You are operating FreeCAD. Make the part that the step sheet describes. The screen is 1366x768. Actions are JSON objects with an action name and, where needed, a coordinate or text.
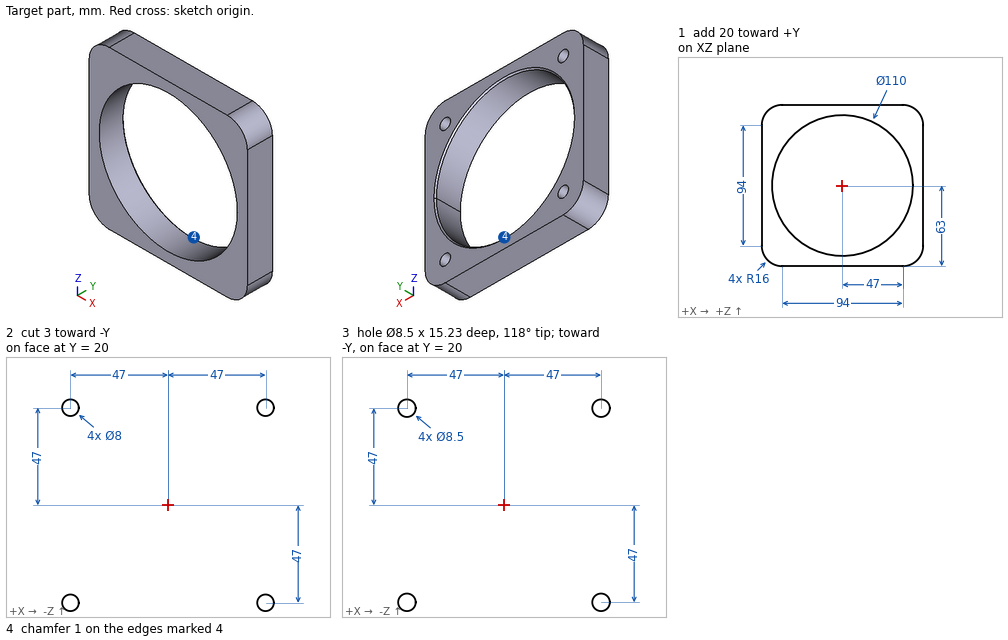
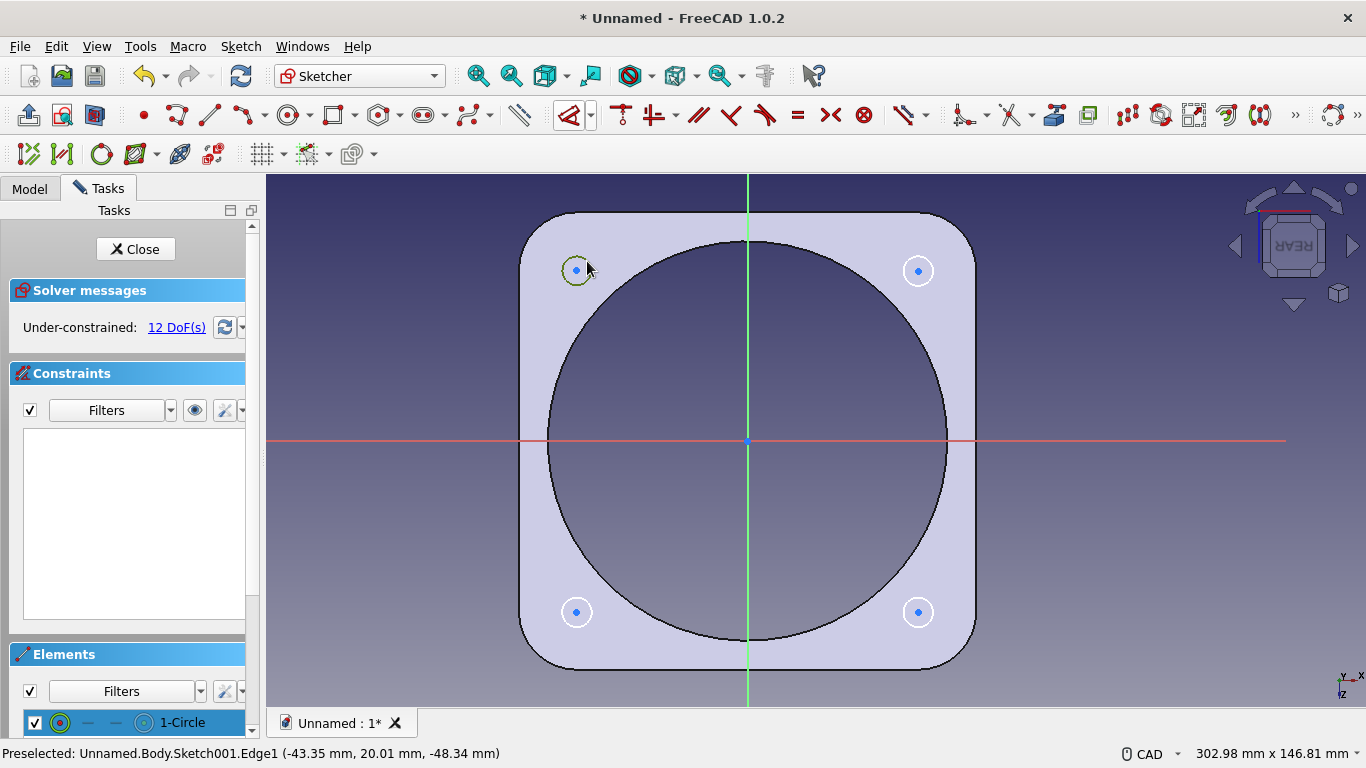
{"action": "left_click", "coordinate": [929, 261]}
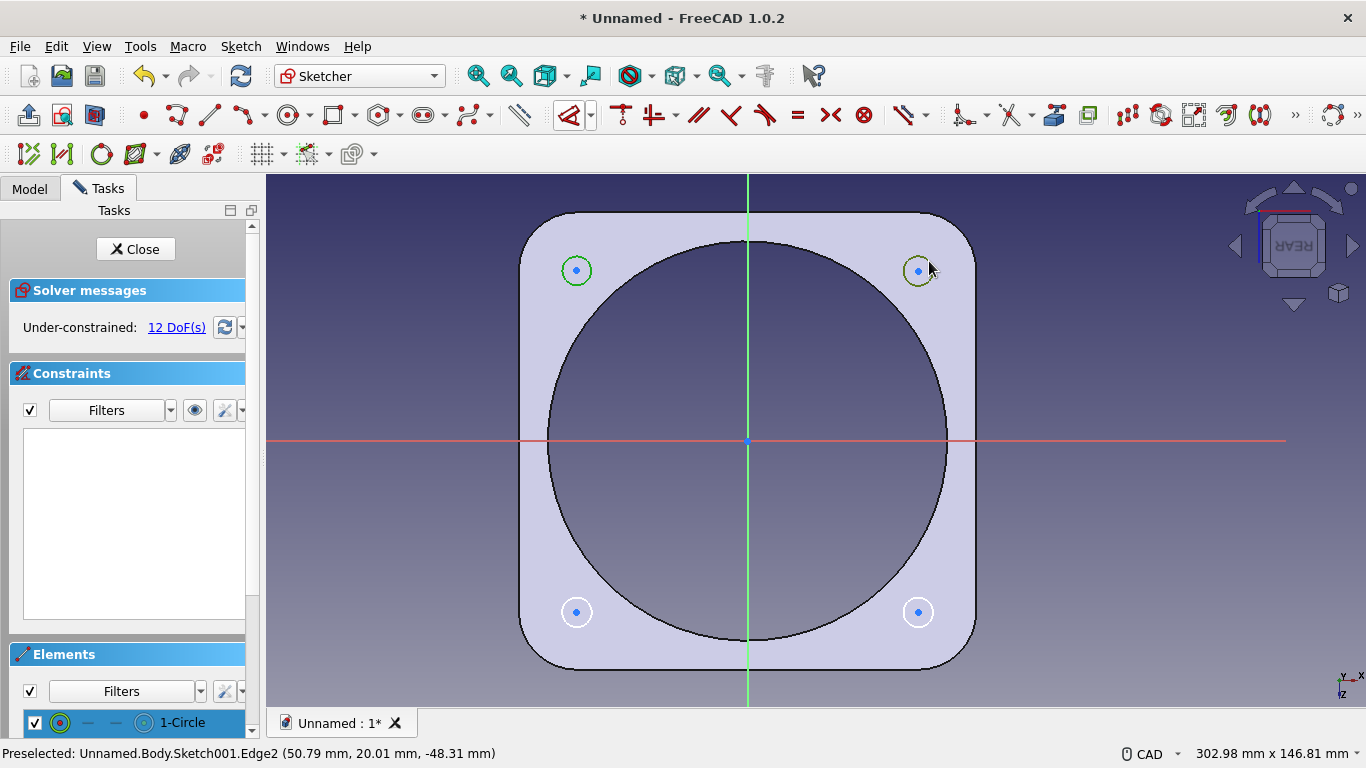
{"action": "left_click", "coordinate": [929, 602]}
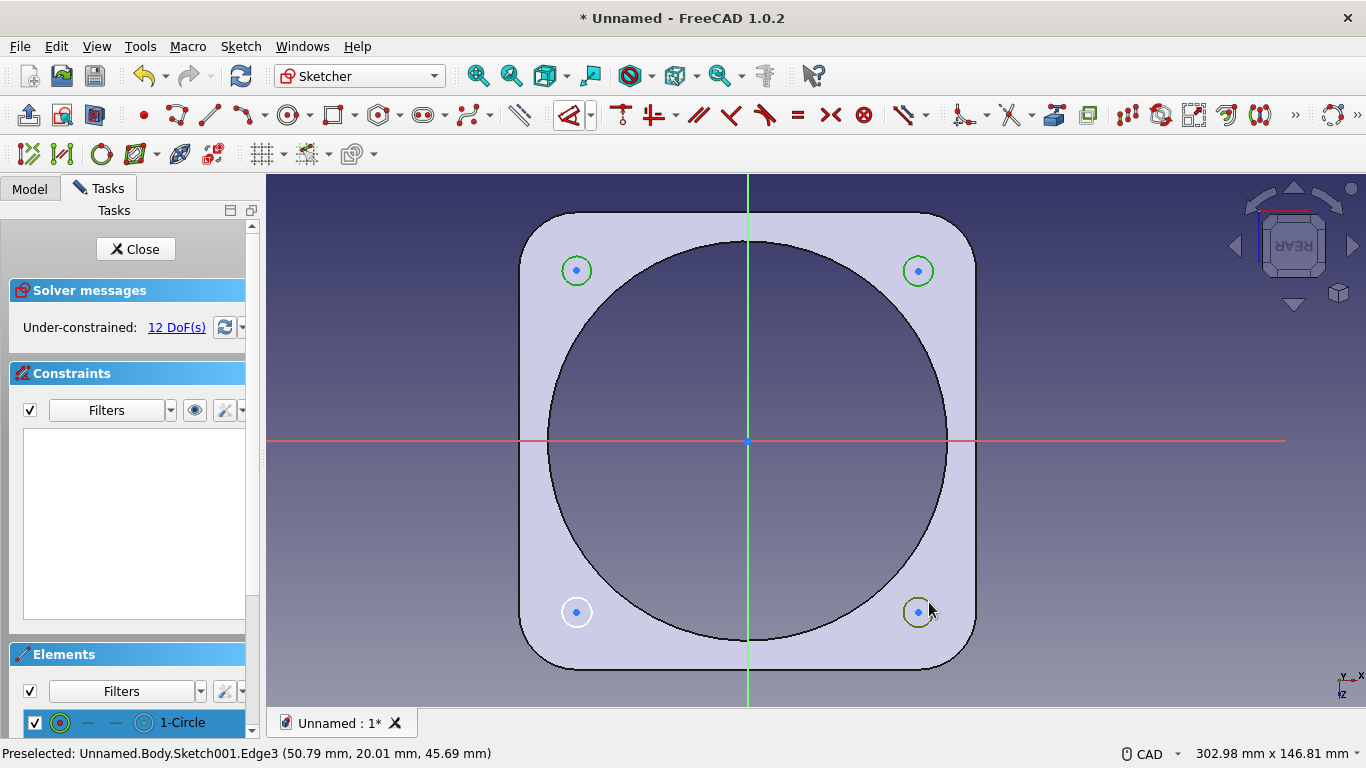
{"action": "left_click", "coordinate": [587, 602]}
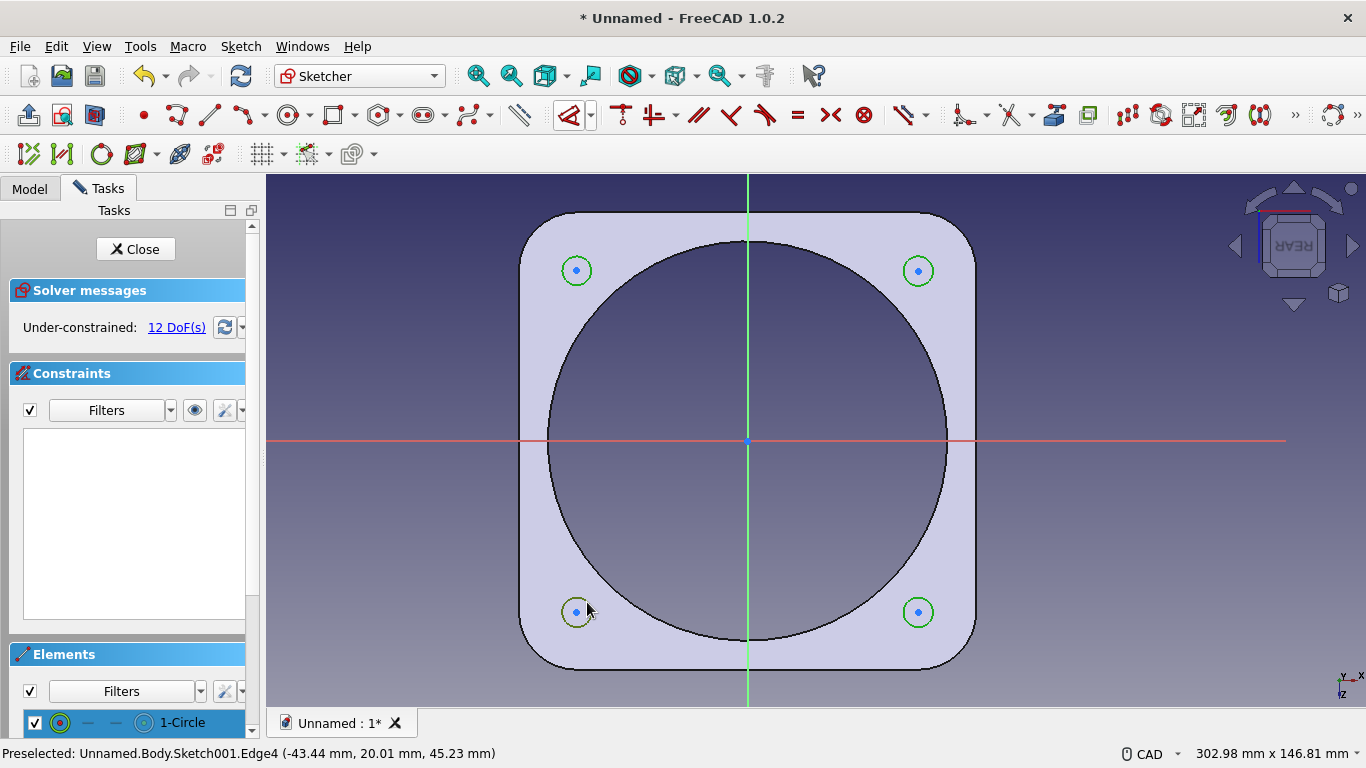
{"action": "left_click", "coordinate": [798, 116]}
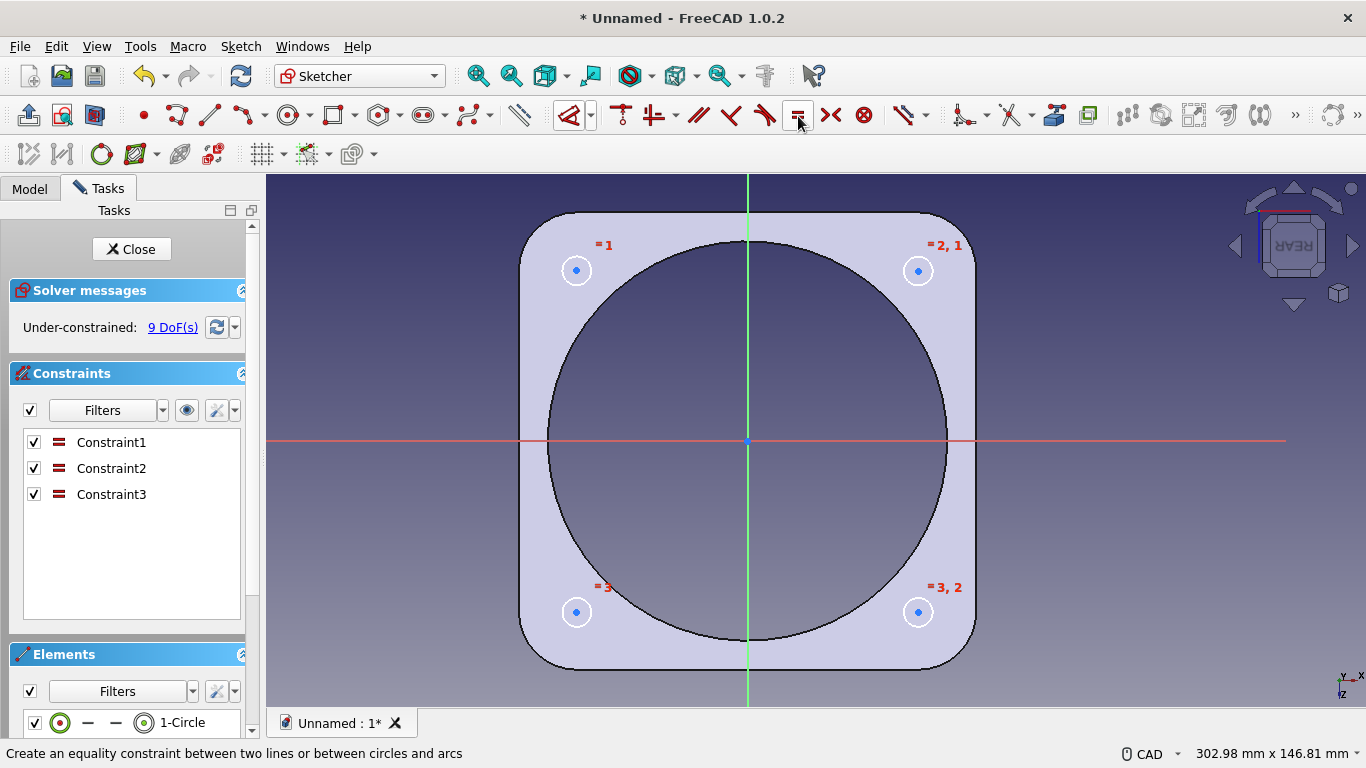
{"action": "left_click", "coordinate": [577, 271]}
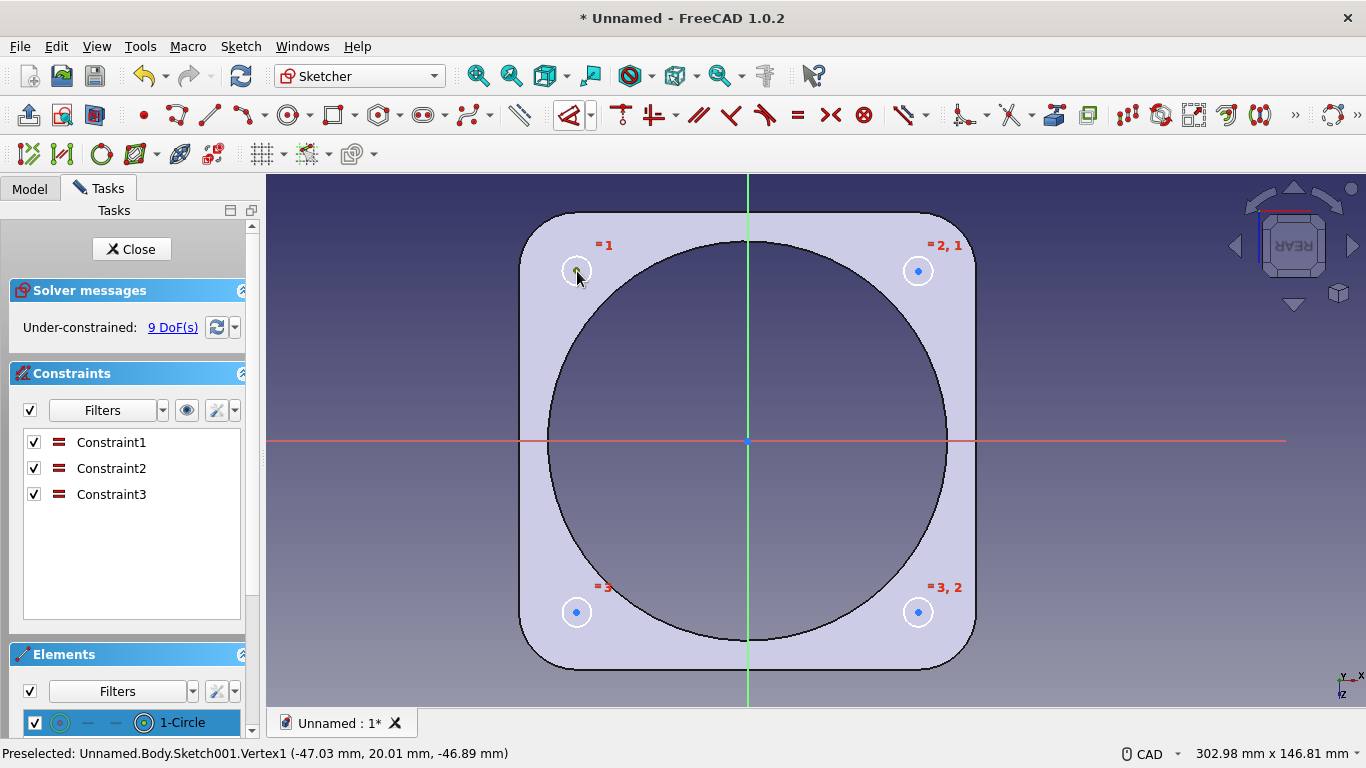
{"action": "left_click", "coordinate": [918, 271]}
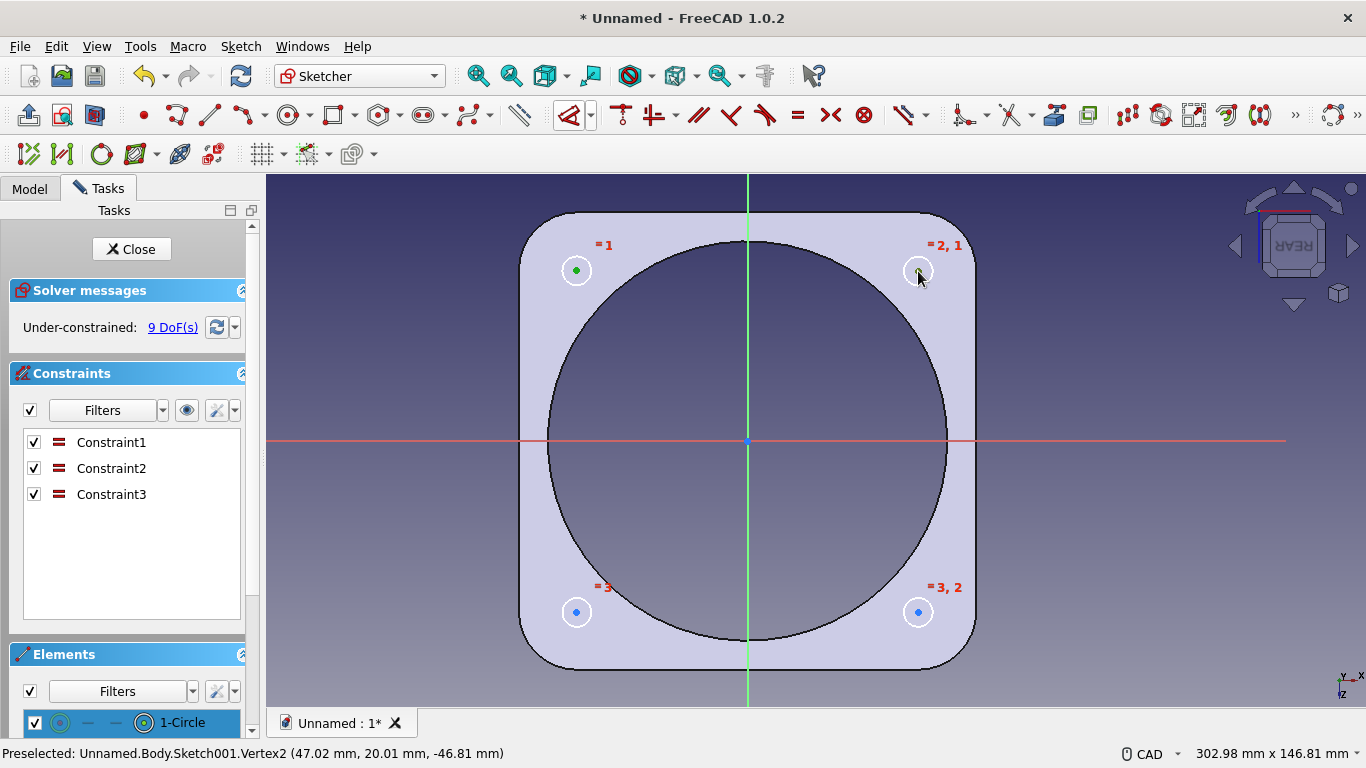
{"action": "key", "text": "h"}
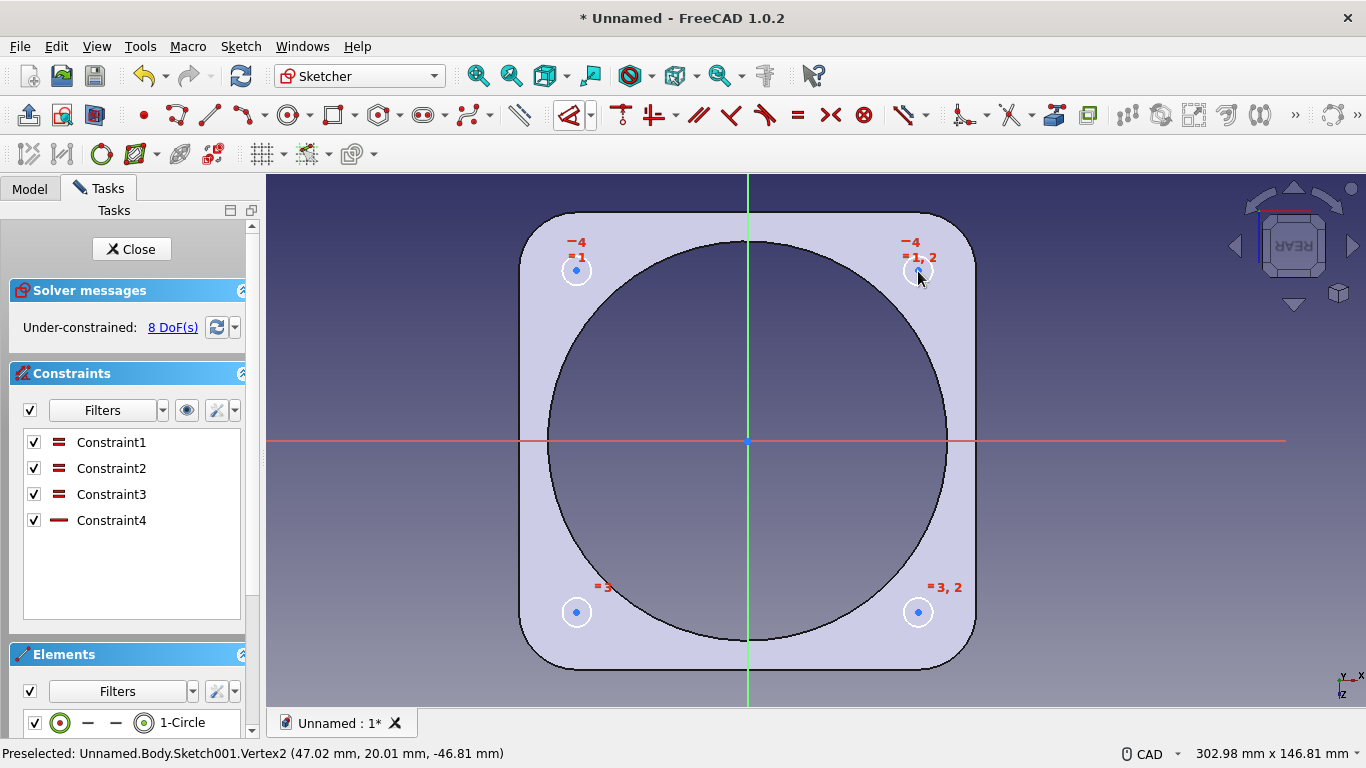
{"action": "left_click", "coordinate": [918, 271]}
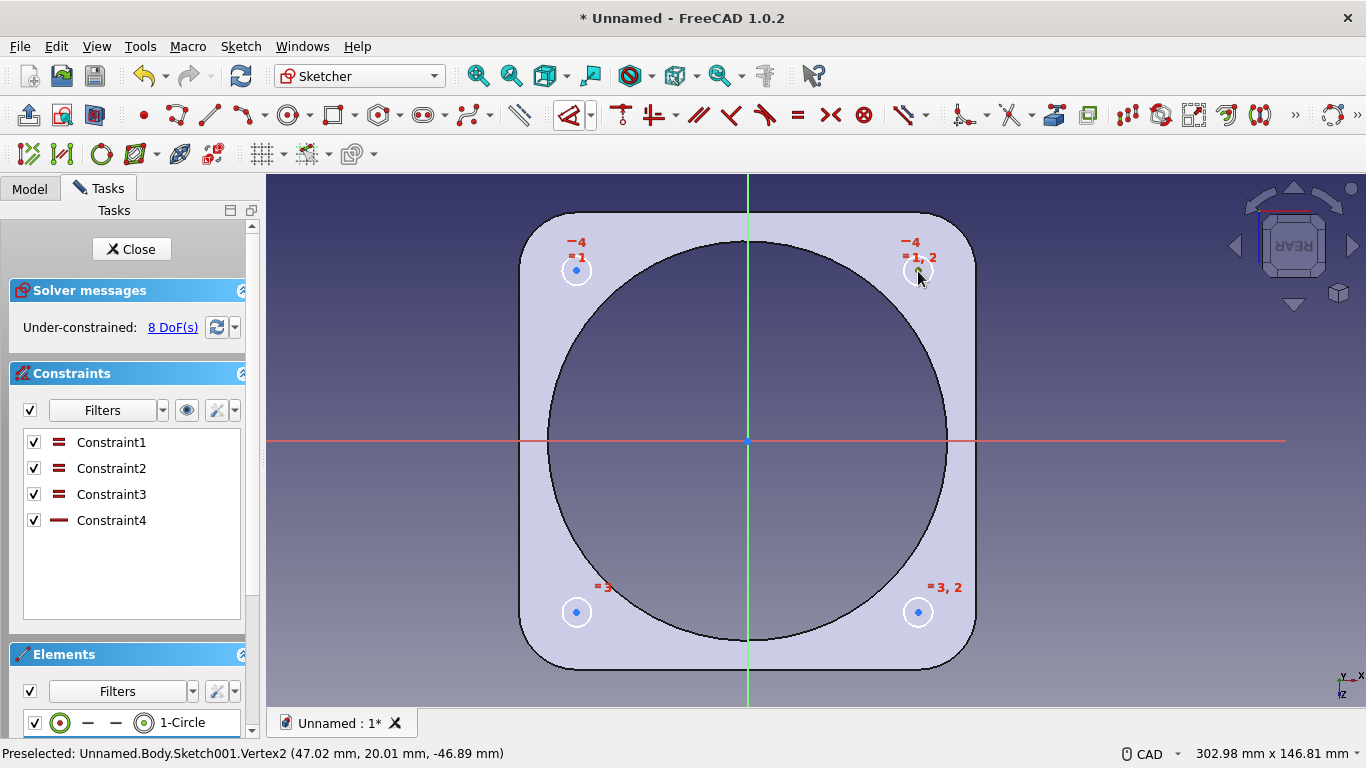
{"action": "left_click", "coordinate": [918, 612]}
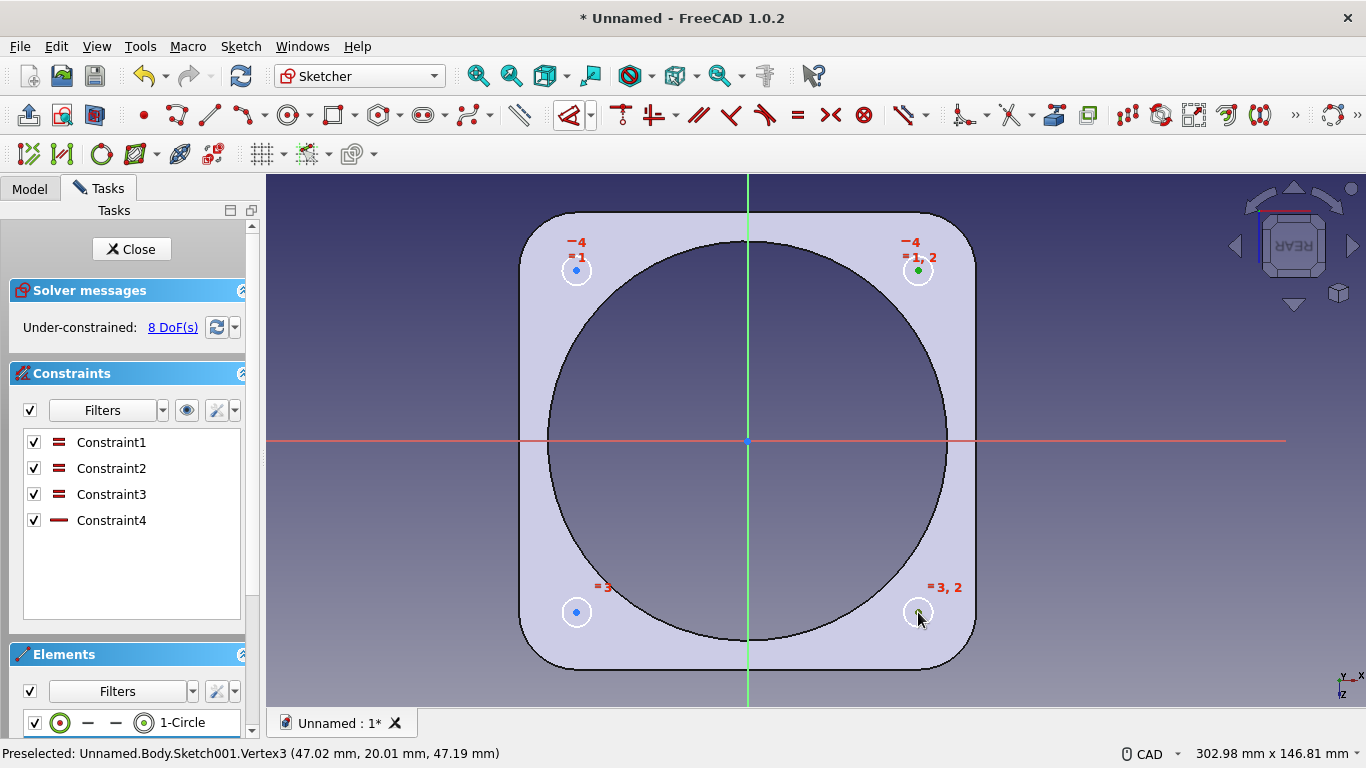
{"action": "left_click", "coordinate": [676, 116]}